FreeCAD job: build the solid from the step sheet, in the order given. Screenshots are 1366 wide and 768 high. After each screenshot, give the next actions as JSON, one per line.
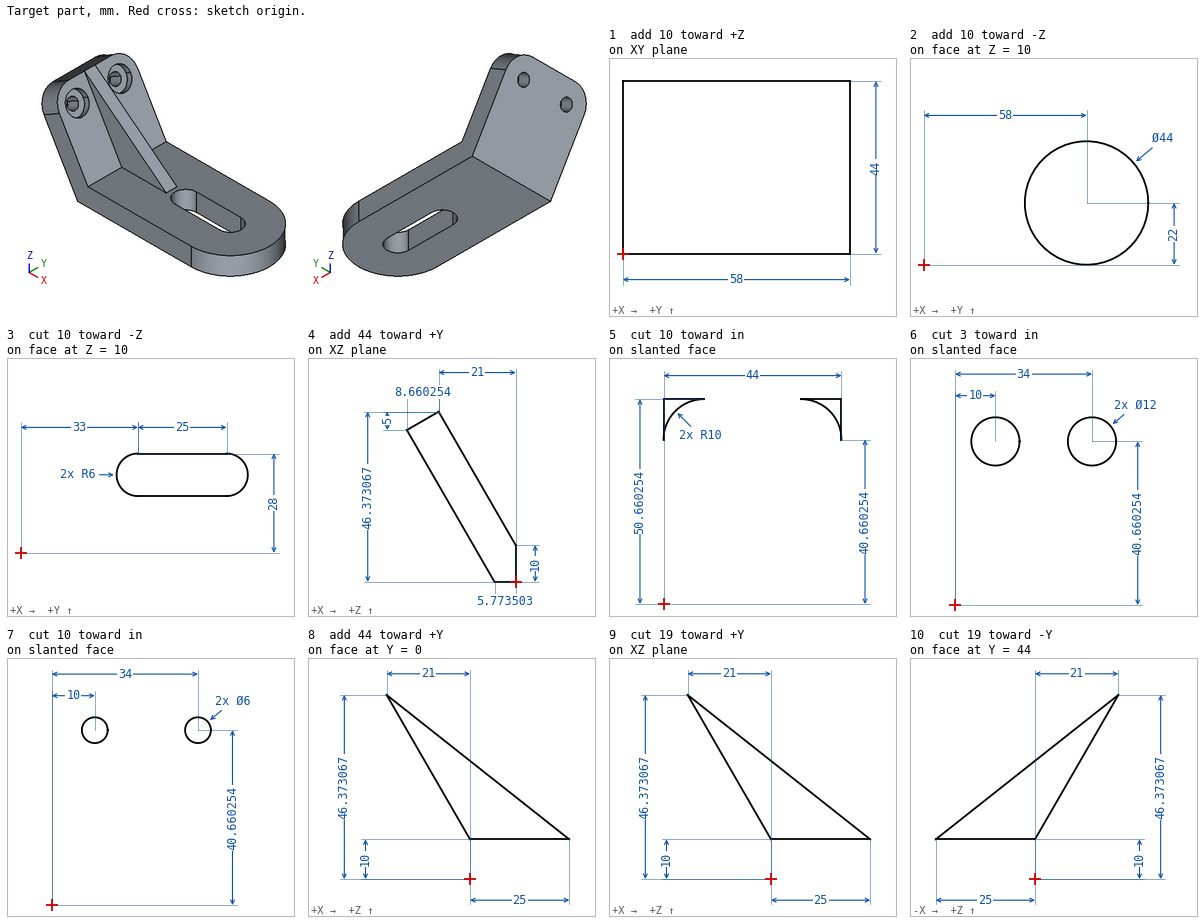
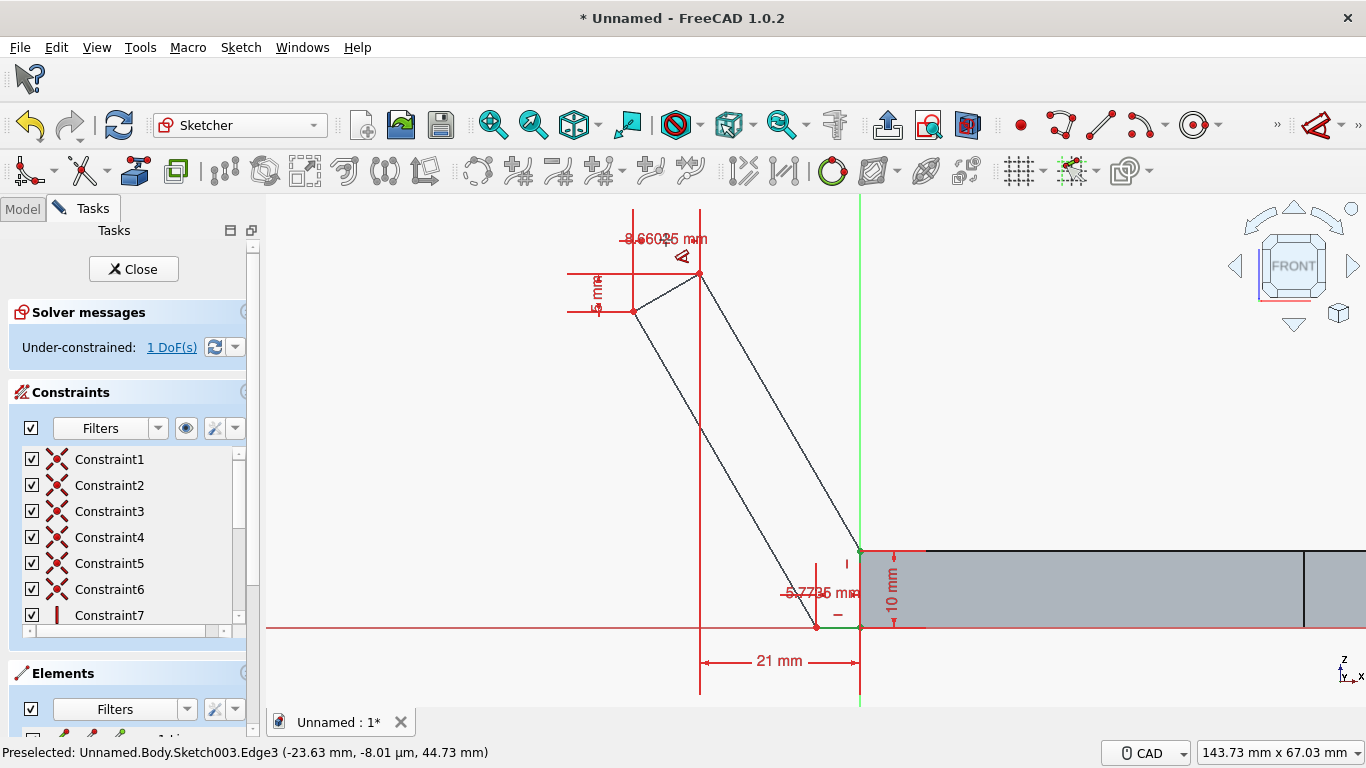
{"action": "left_click", "coordinate": [700, 274]}
{"action": "left_click", "coordinate": [894, 451]}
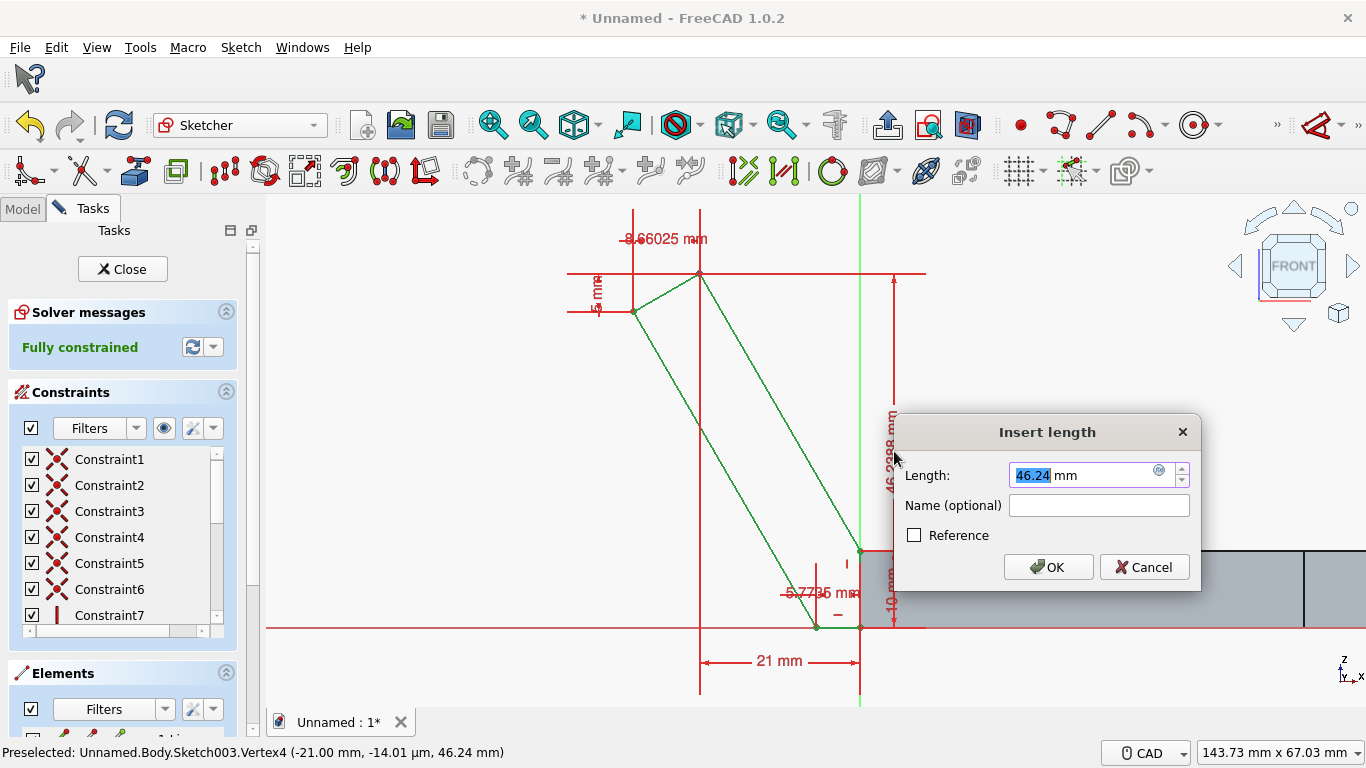
{"action": "type", "text": "46.373067"}
{"action": "key", "text": "Return"}
{"action": "key", "text": "Escape"}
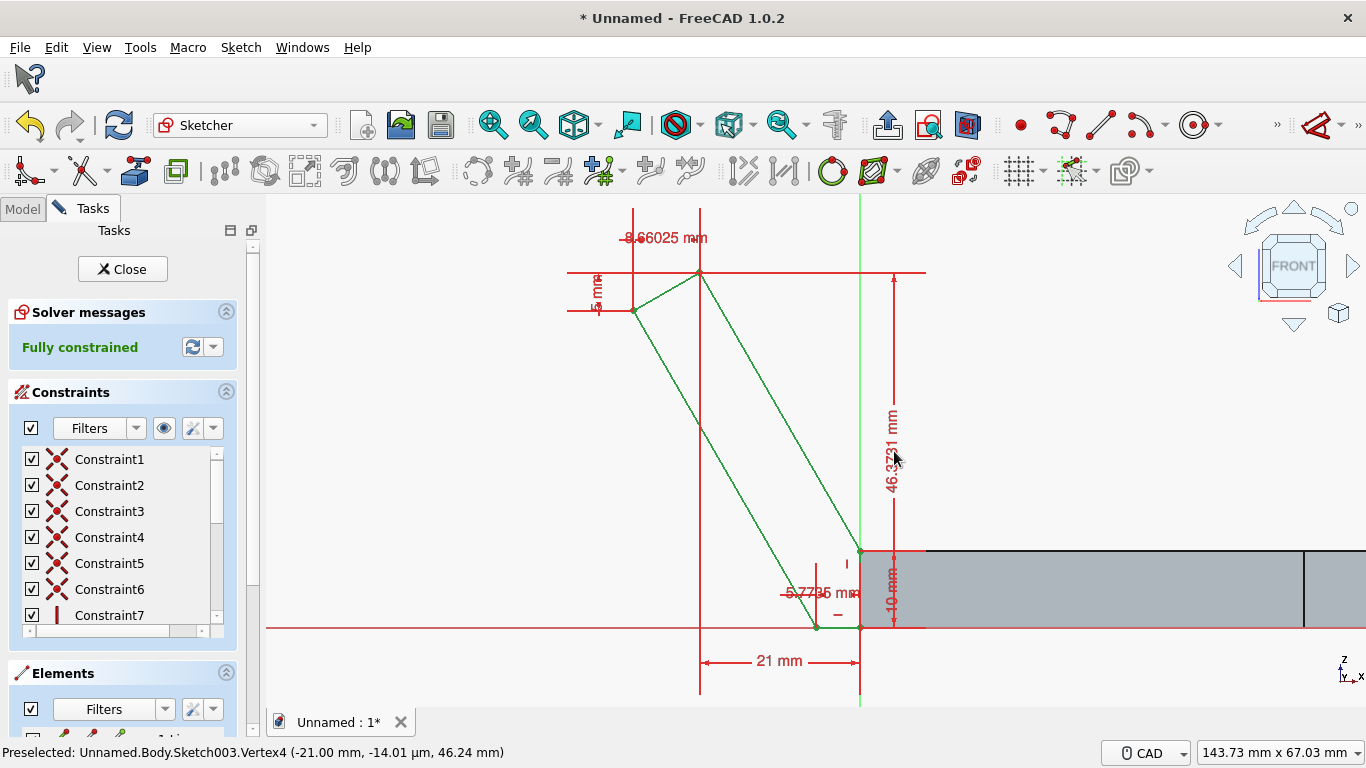
{"action": "left_click", "coordinate": [123, 269]}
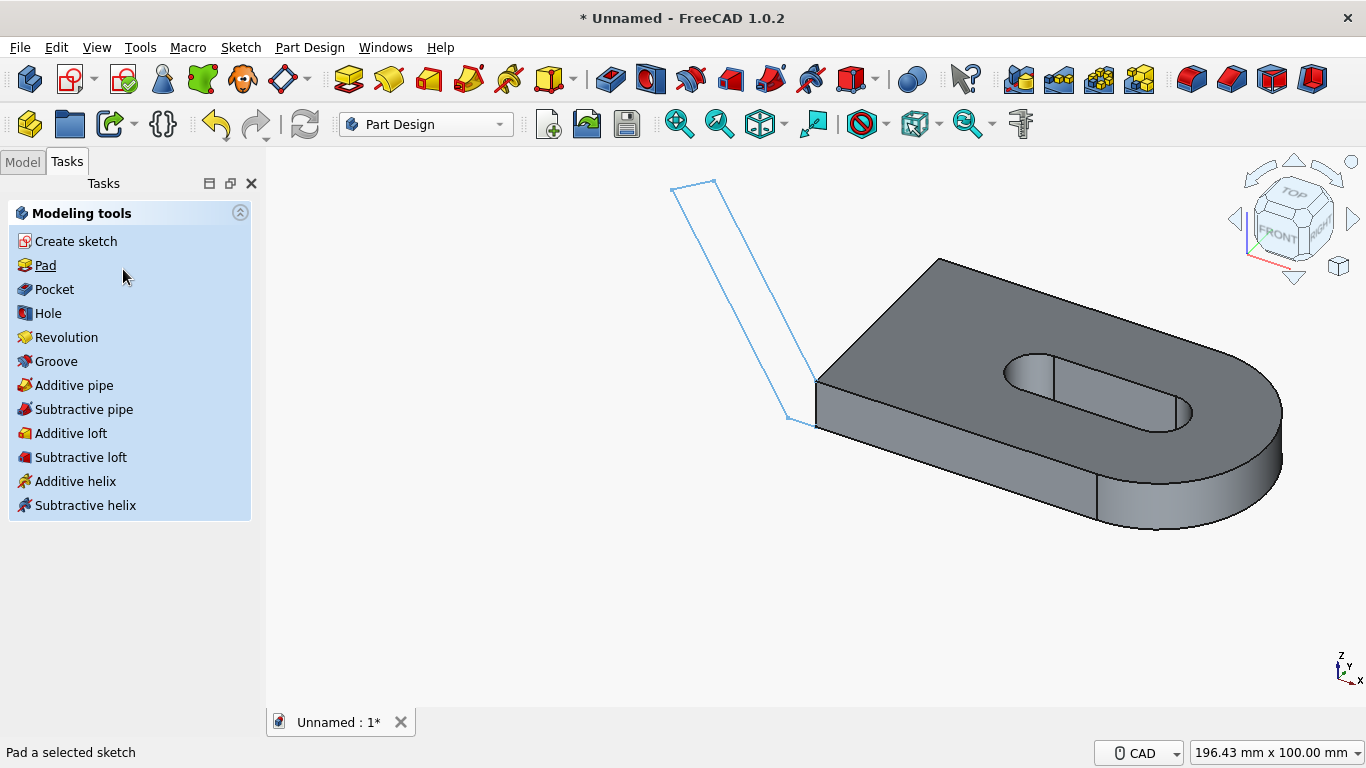
{"action": "left_click", "coordinate": [350, 80]}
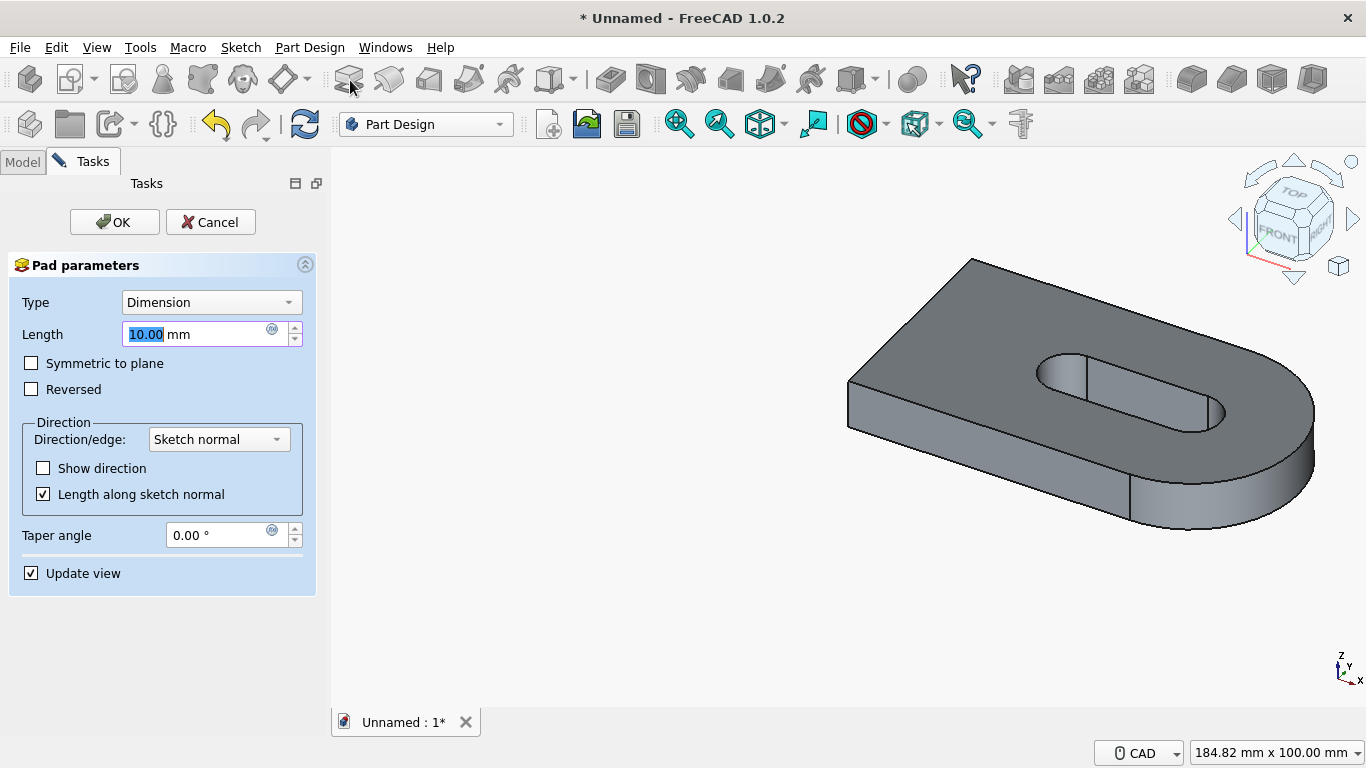
{"action": "type", "text": "44"}
{"action": "key", "text": "Tab"}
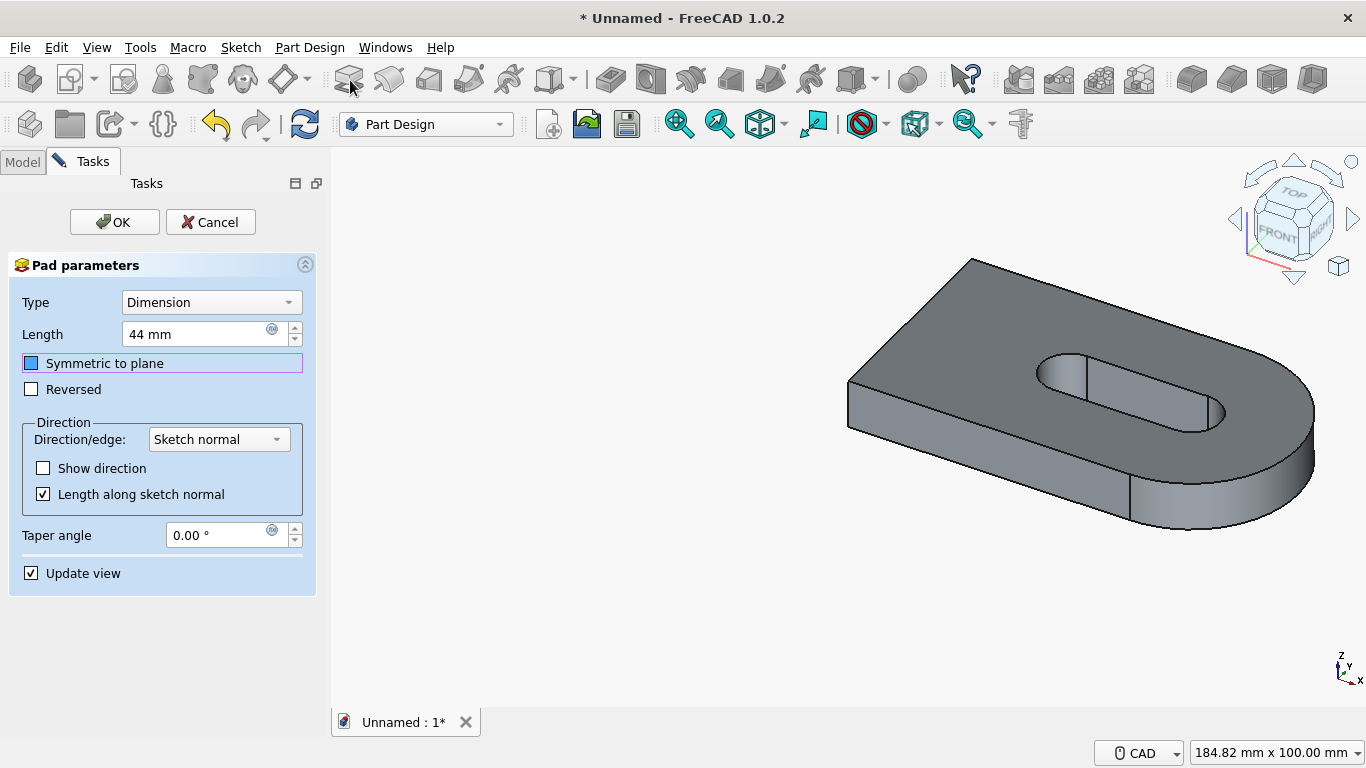
{"action": "left_click", "coordinate": [30, 389]}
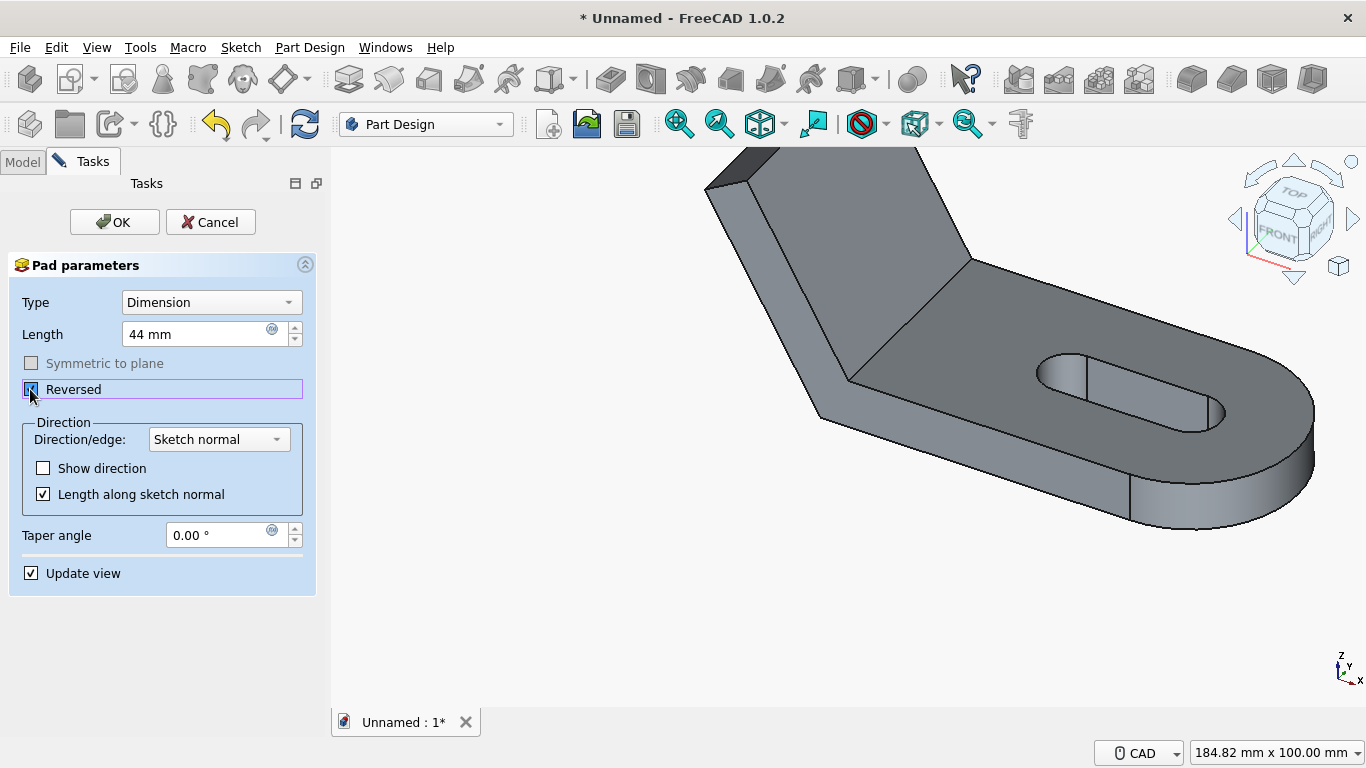
{"action": "left_click", "coordinate": [115, 222]}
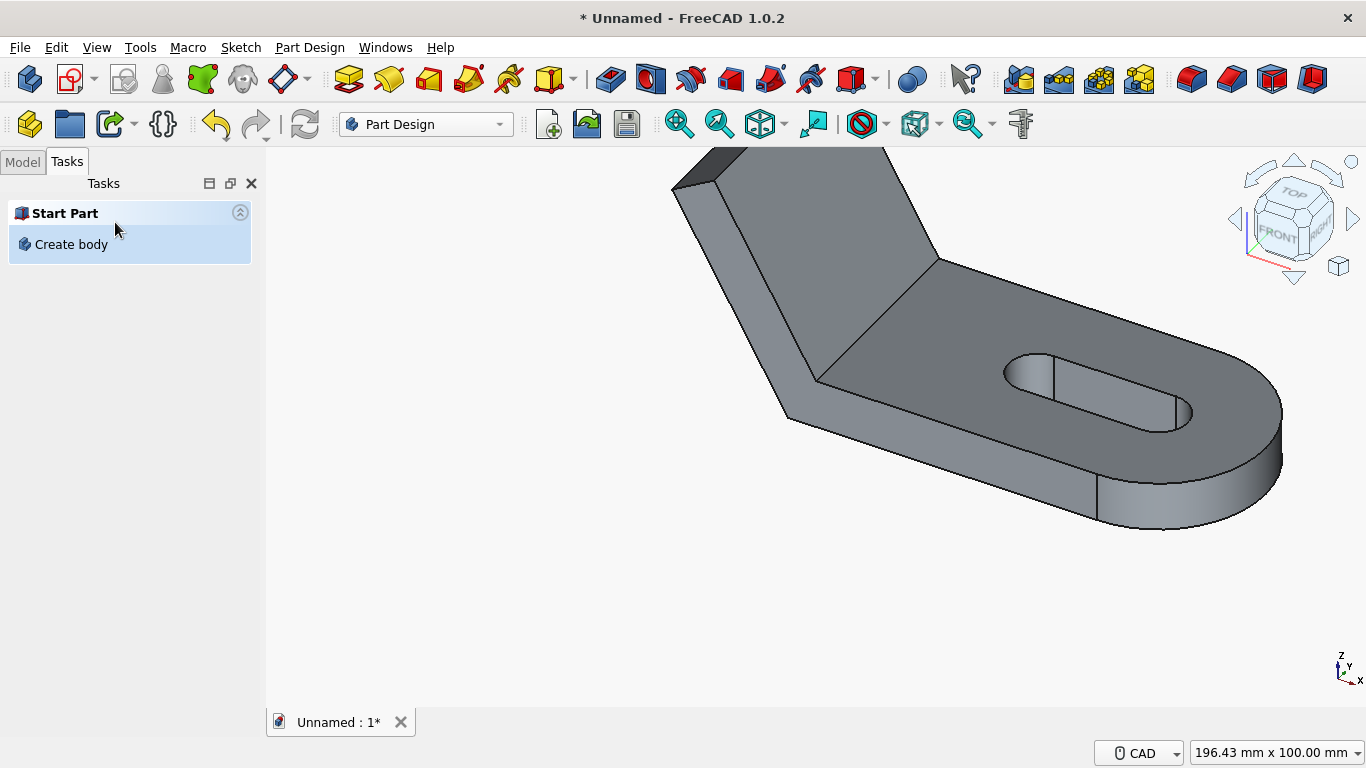
{"action": "left_click", "coordinate": [680, 124]}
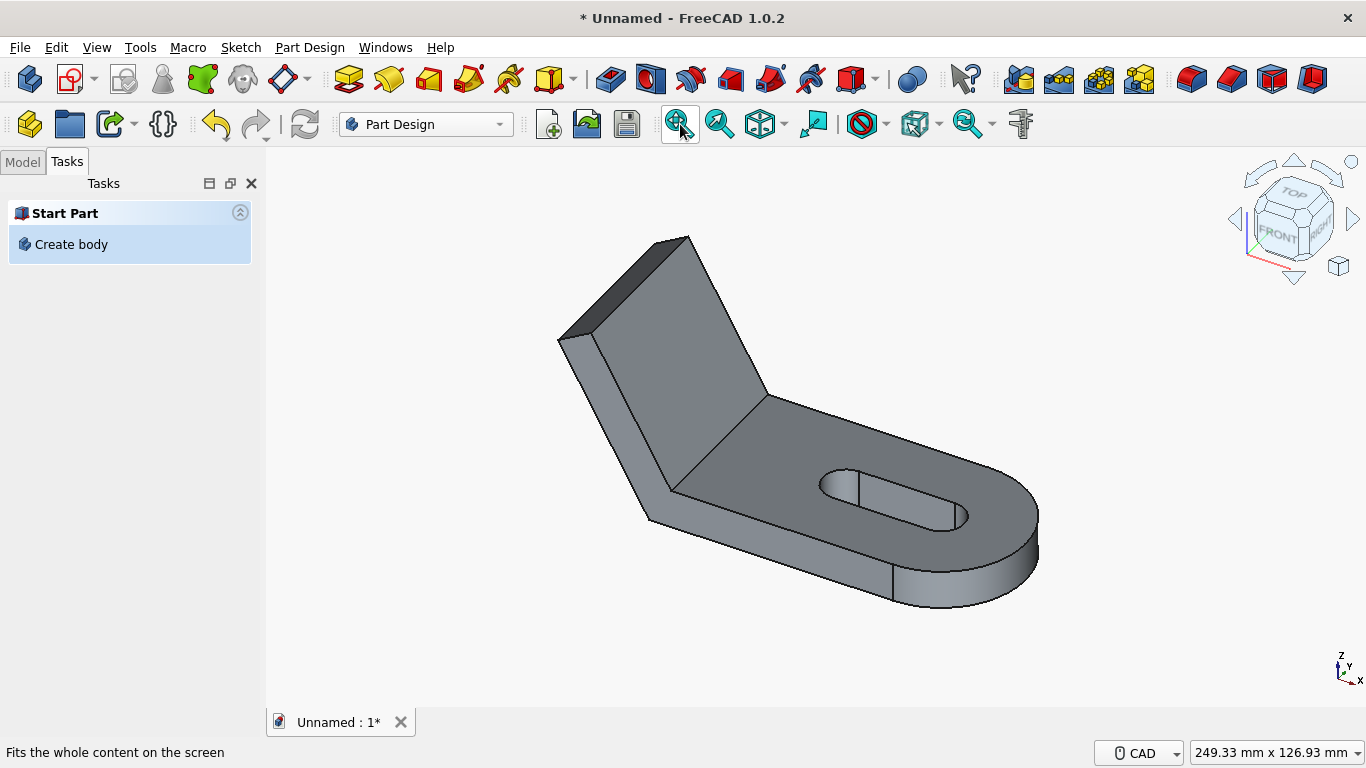
{"action": "left_click", "coordinate": [680, 363]}